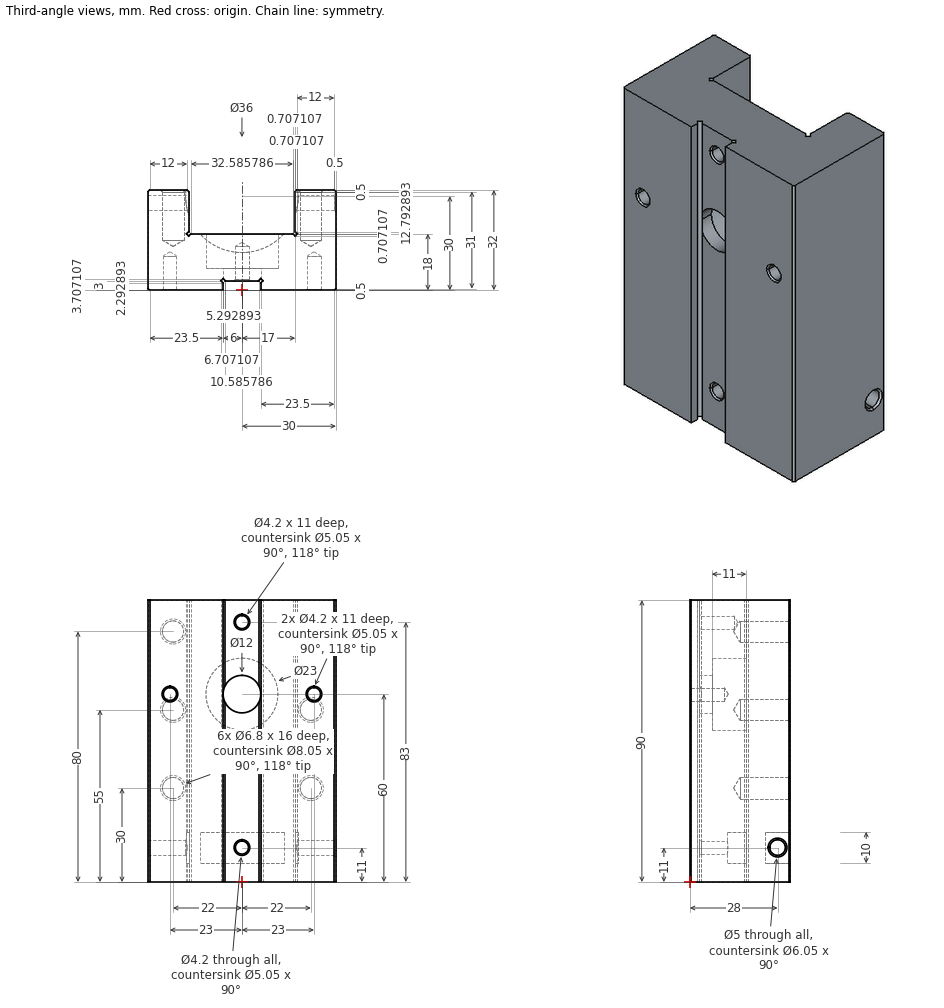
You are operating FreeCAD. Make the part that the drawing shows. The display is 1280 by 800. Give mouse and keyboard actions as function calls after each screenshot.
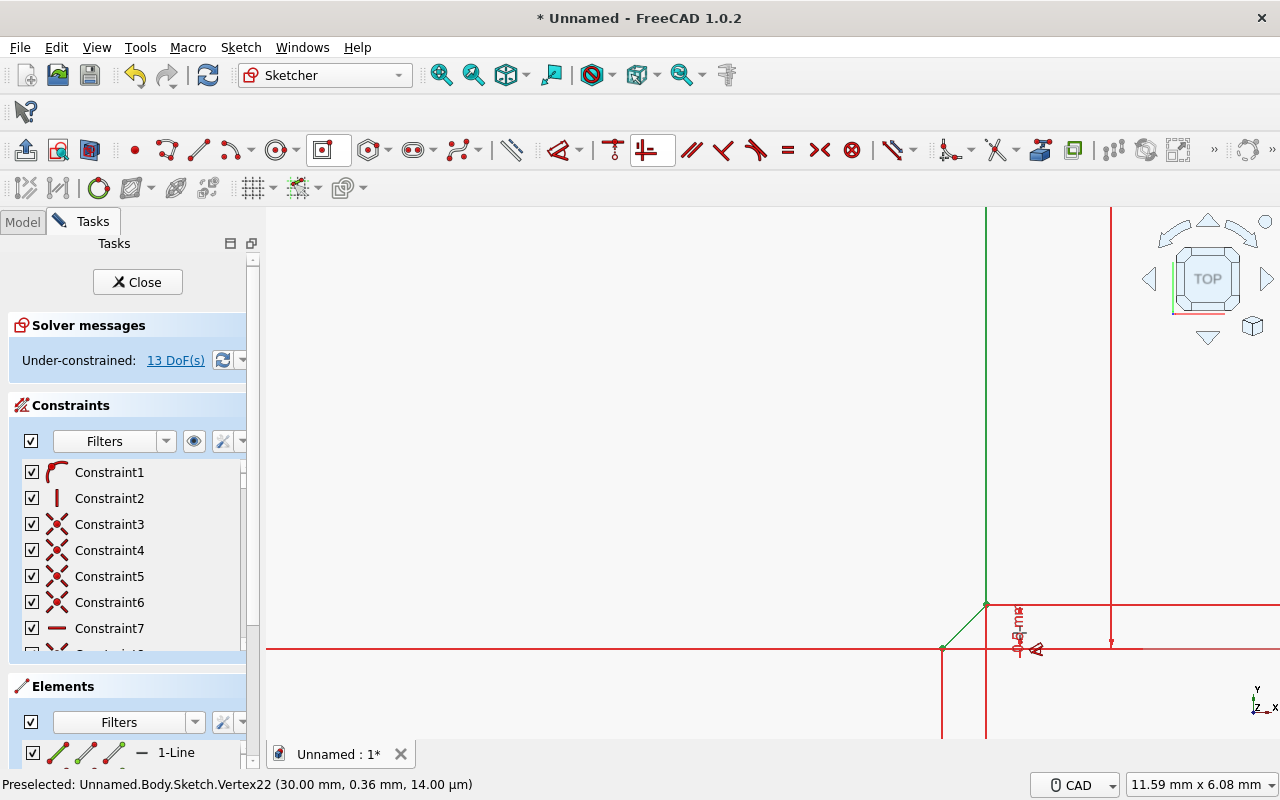
scroll(996, 626, down, 11)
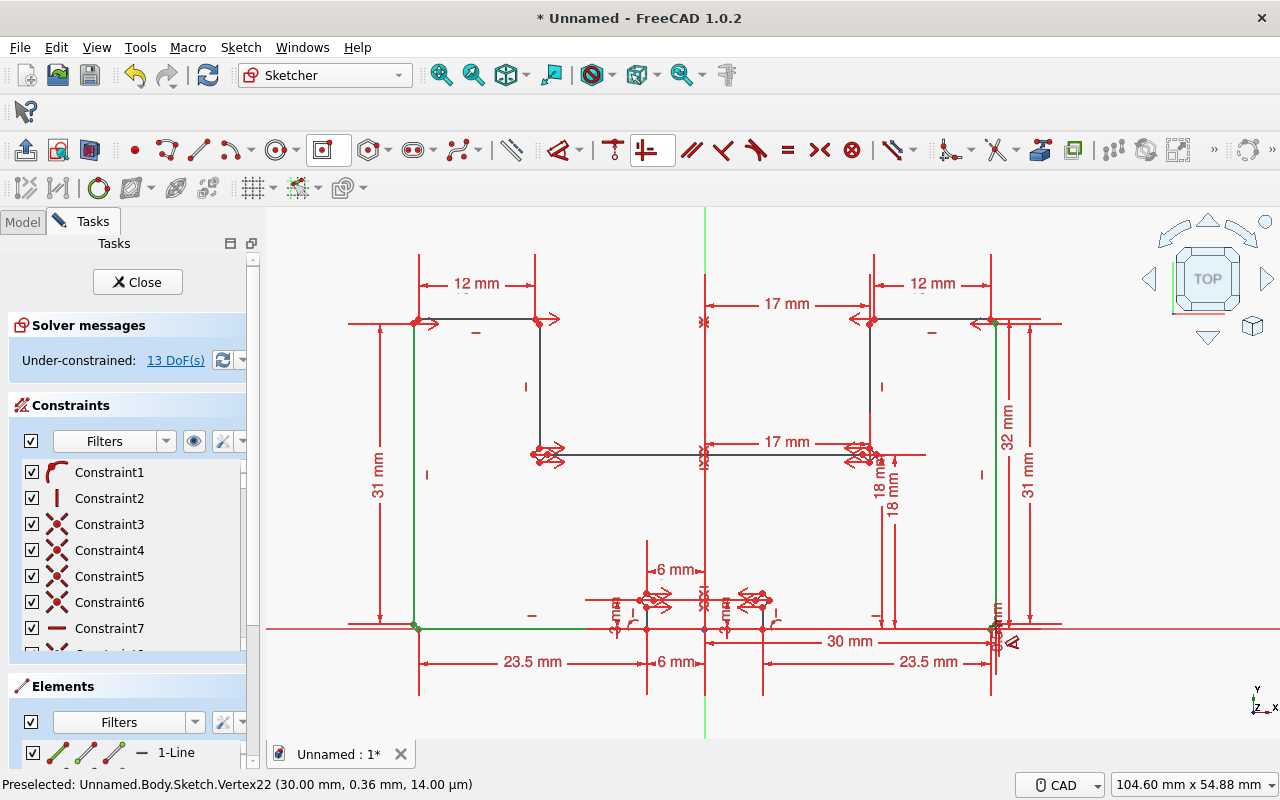
scroll(994, 322, up, 11)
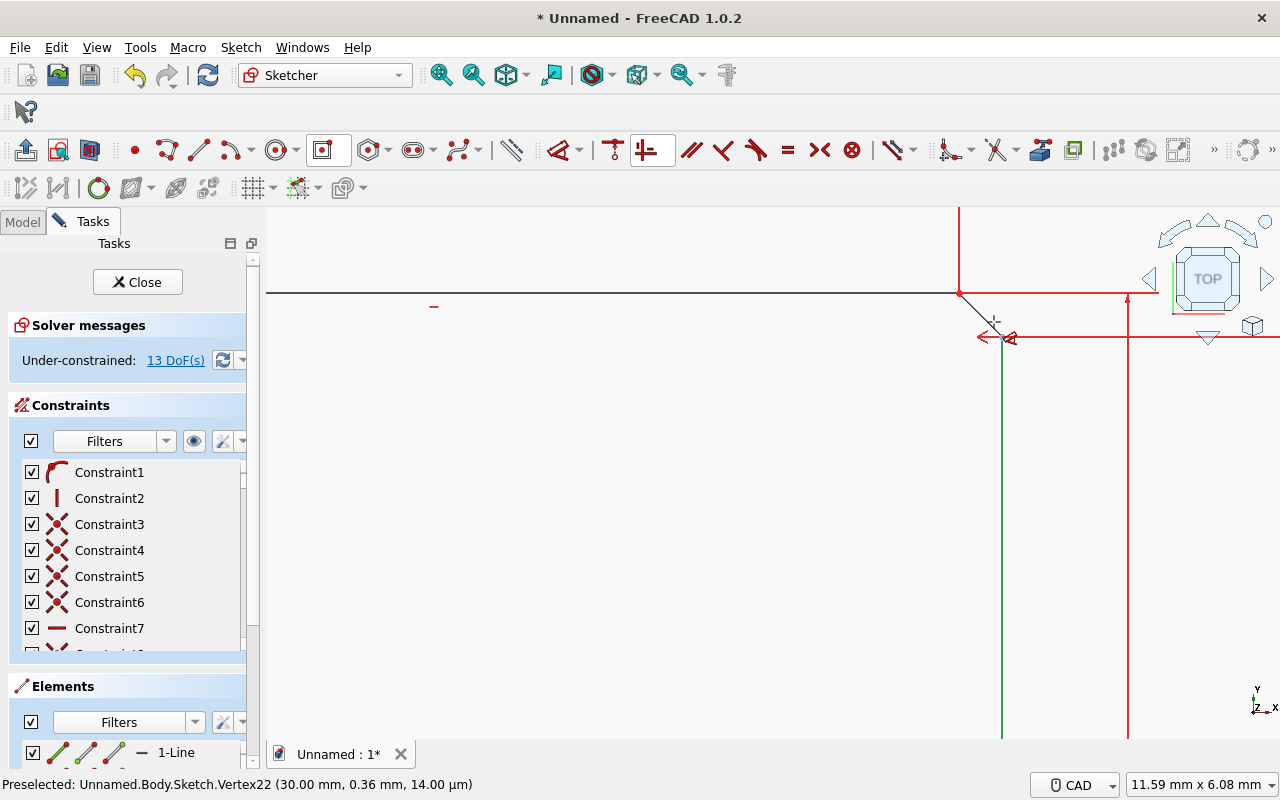
click(989, 324)
click(981, 259)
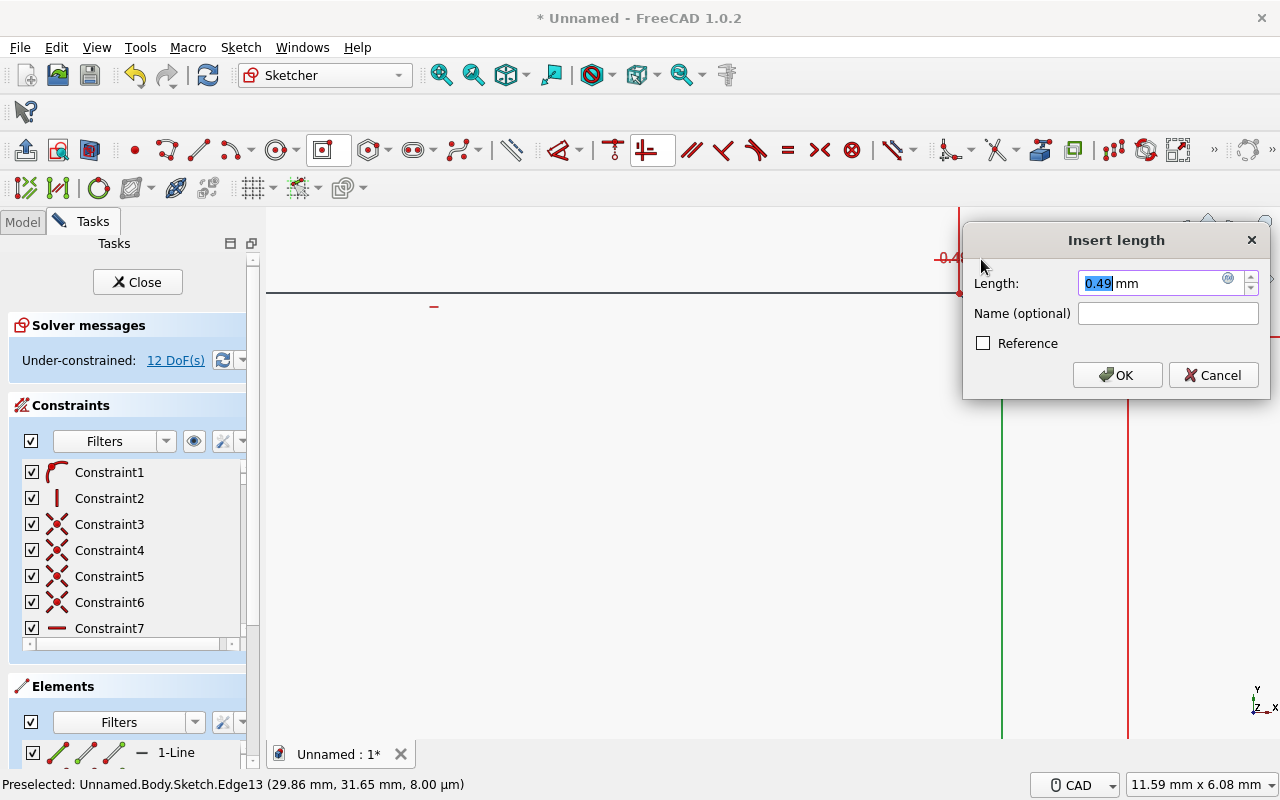
text(0.5)
key(Return)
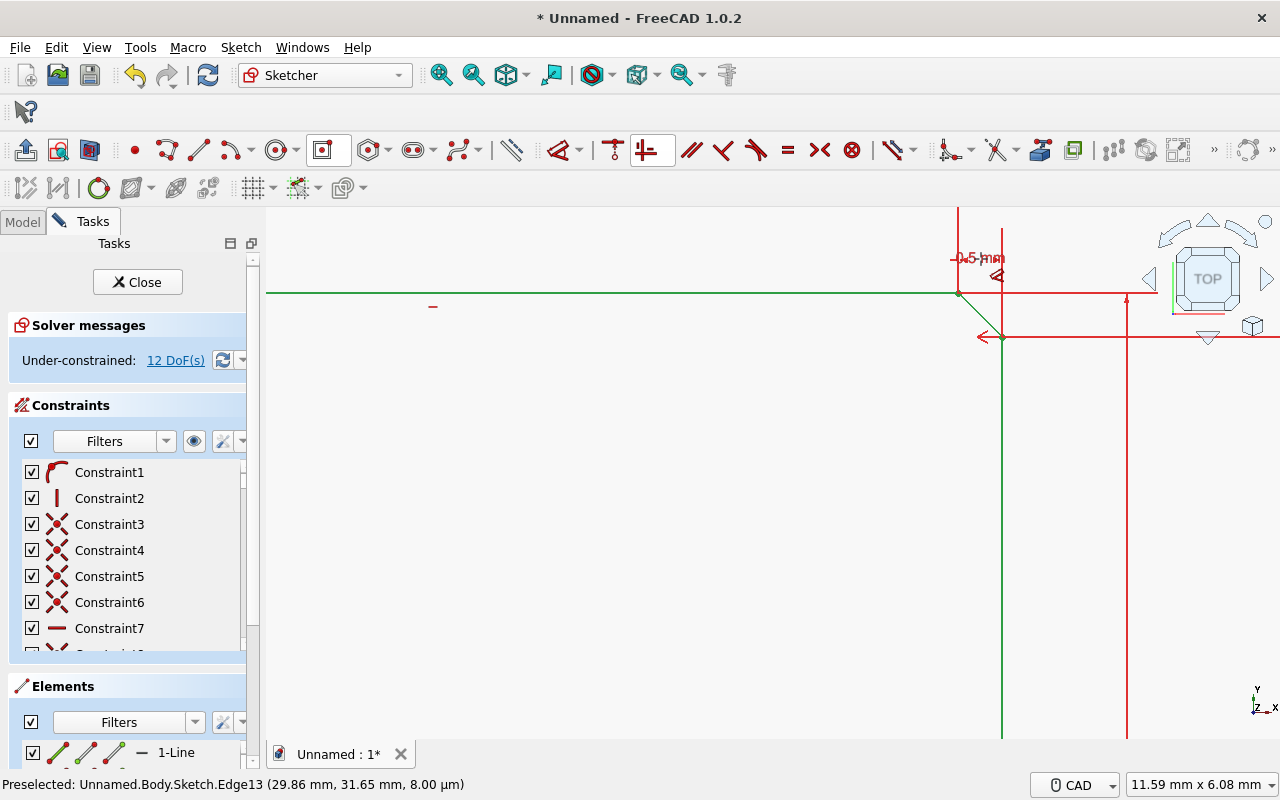
scroll(994, 321, down, 11)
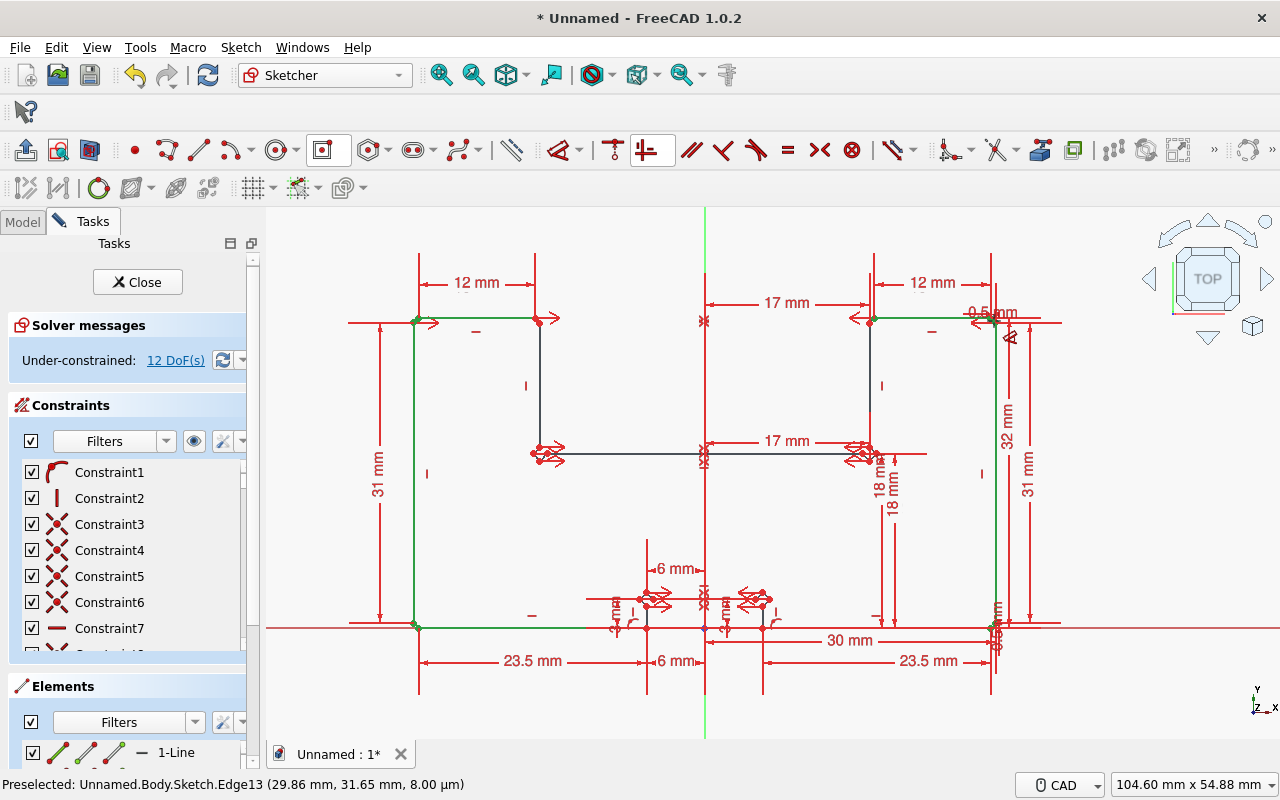
scroll(873, 320, up, 11)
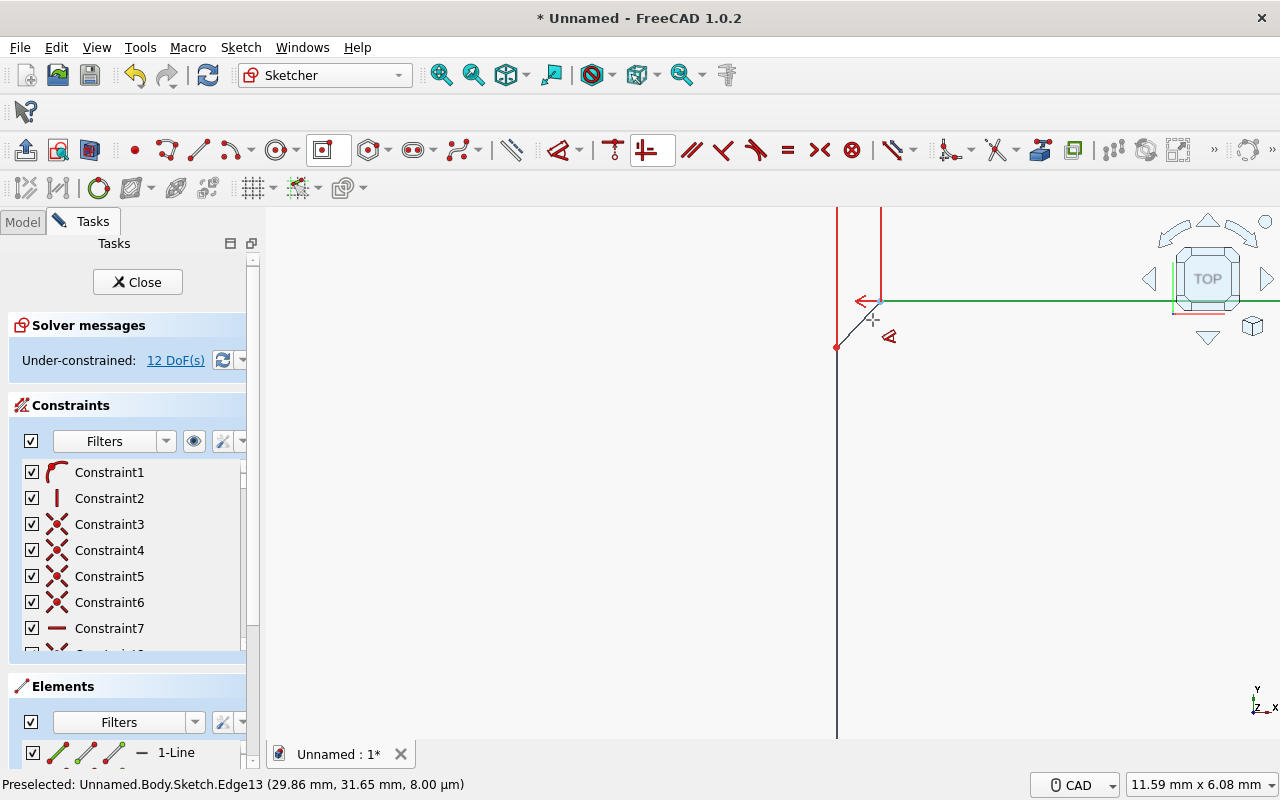
click(867, 315)
click(915, 325)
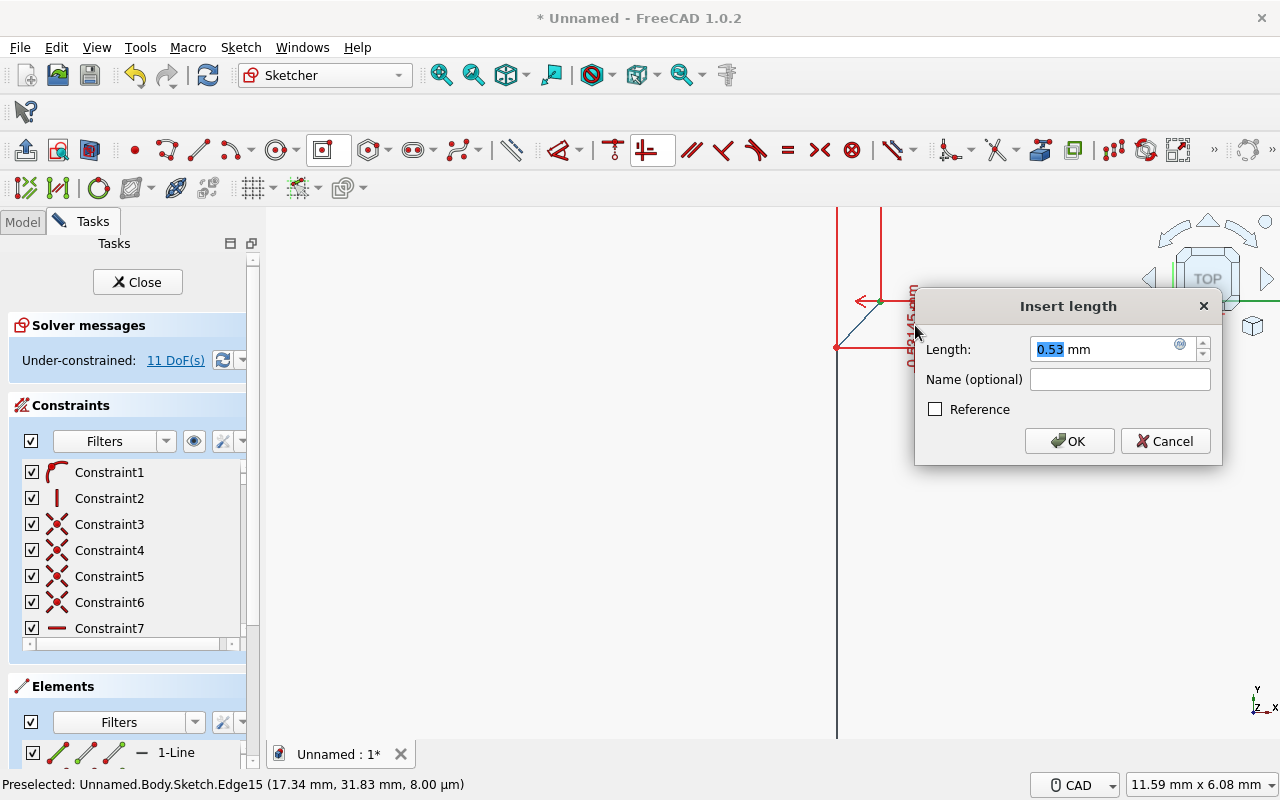
text(0.5)
key(Return)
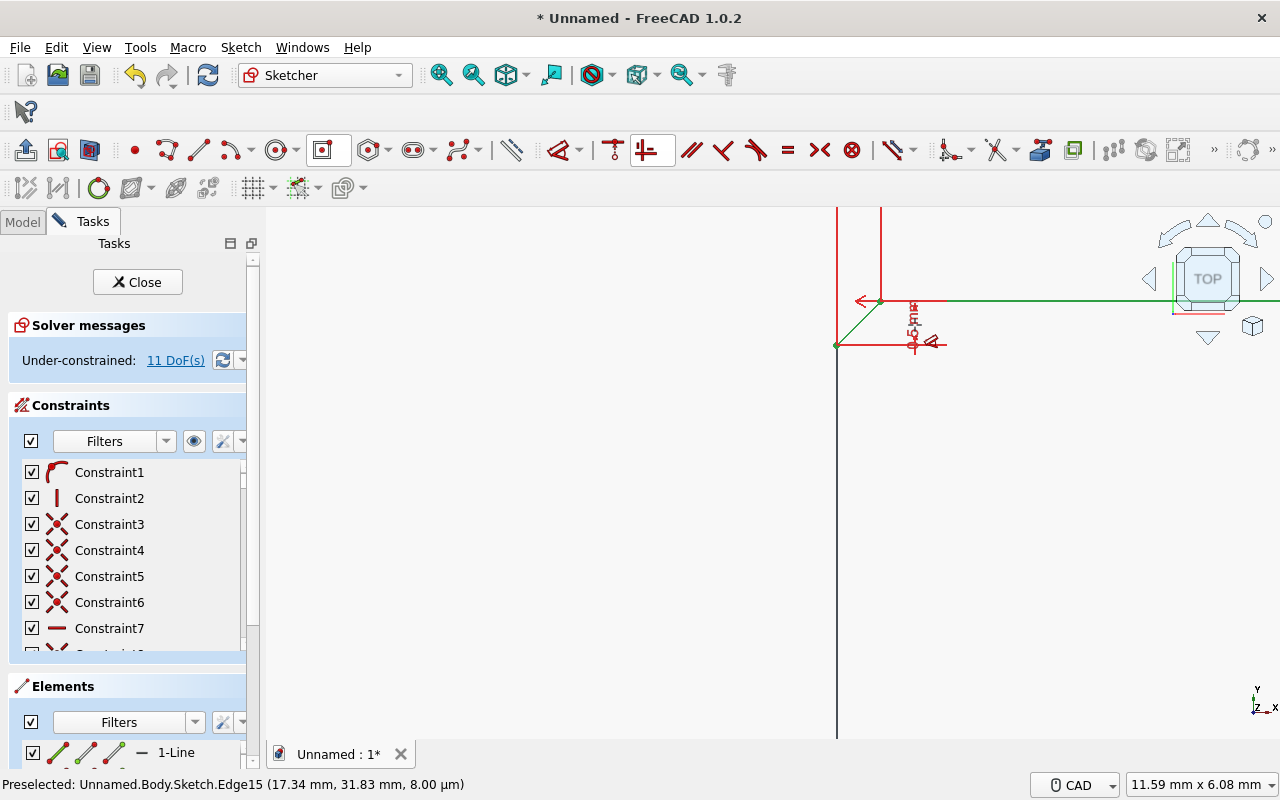
scroll(873, 320, down, 11)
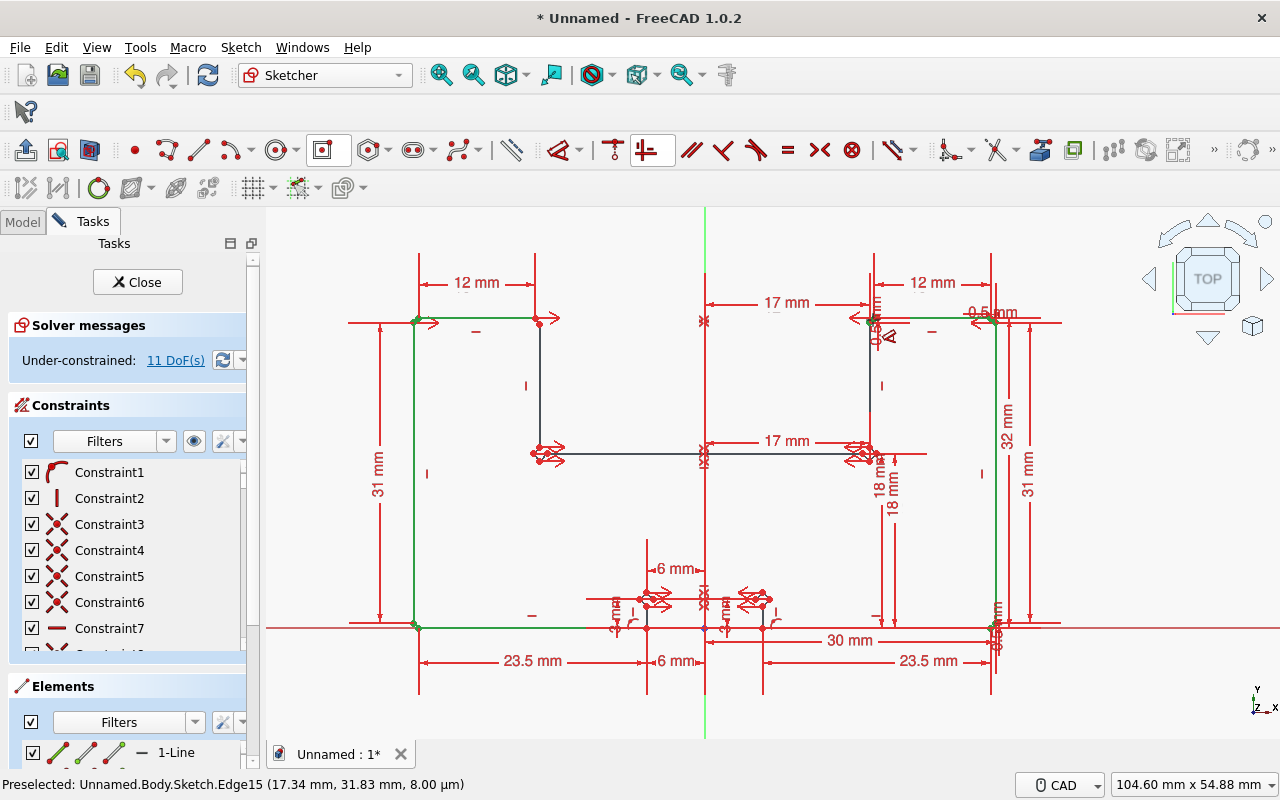
scroll(538, 322, up, 11)